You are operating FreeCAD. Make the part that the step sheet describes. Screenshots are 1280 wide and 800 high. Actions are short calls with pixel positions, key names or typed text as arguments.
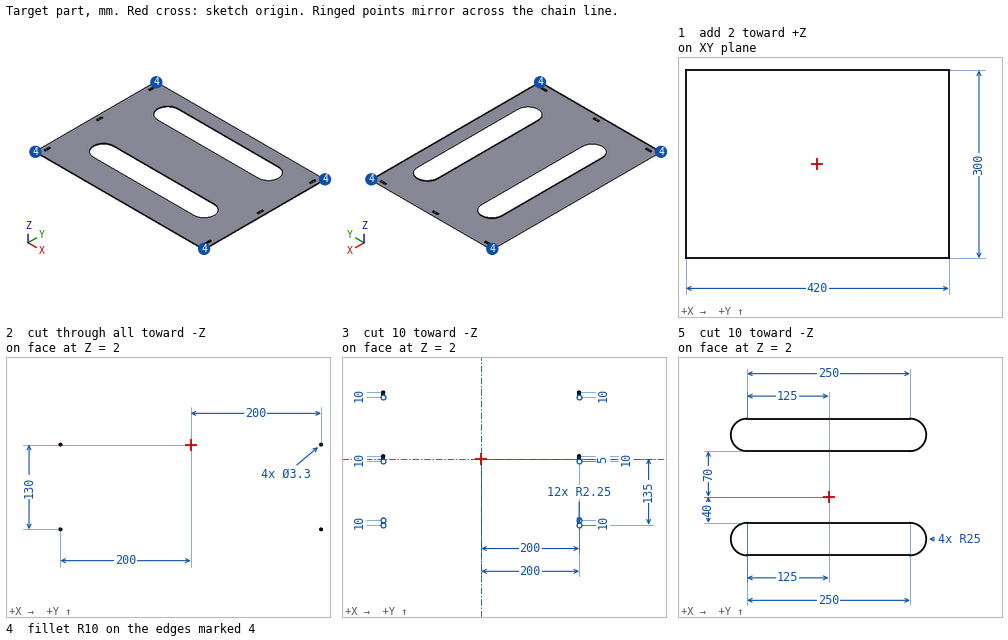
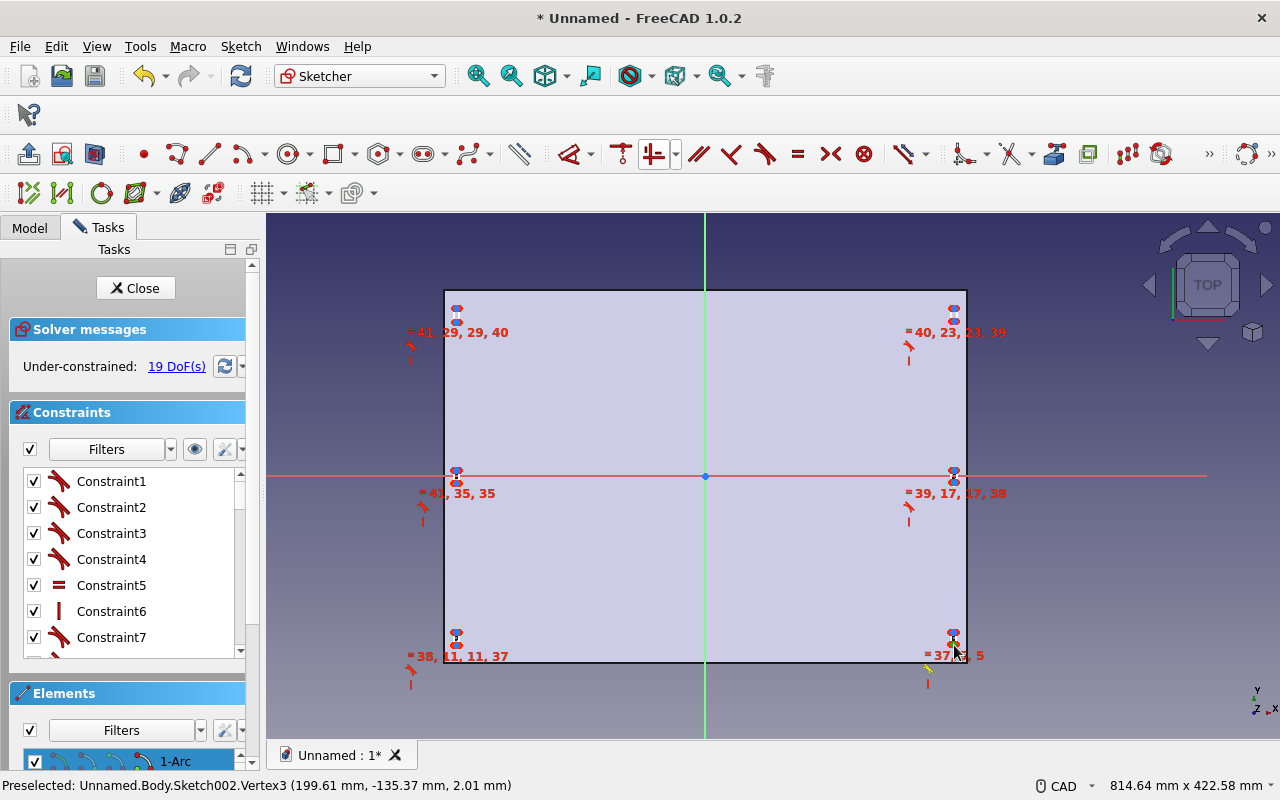
scroll(456, 645, up, 8)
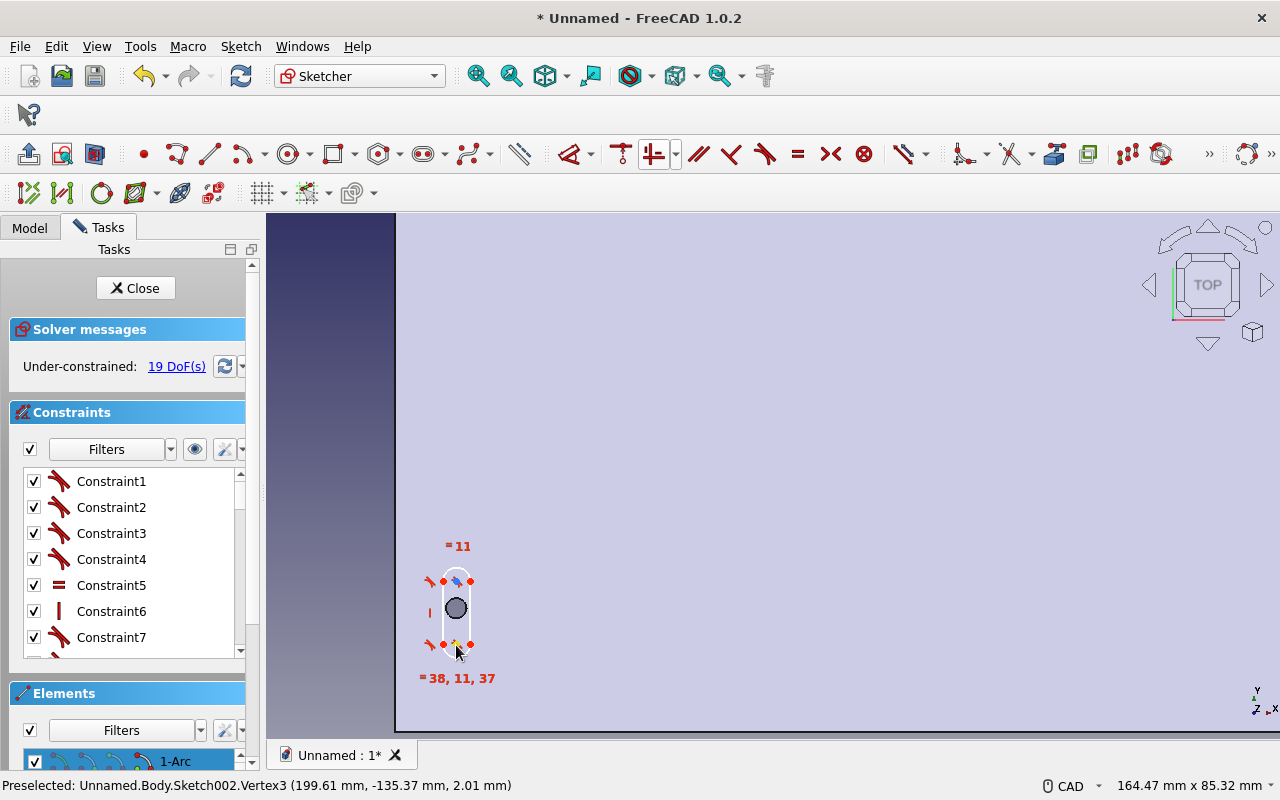
click(457, 644)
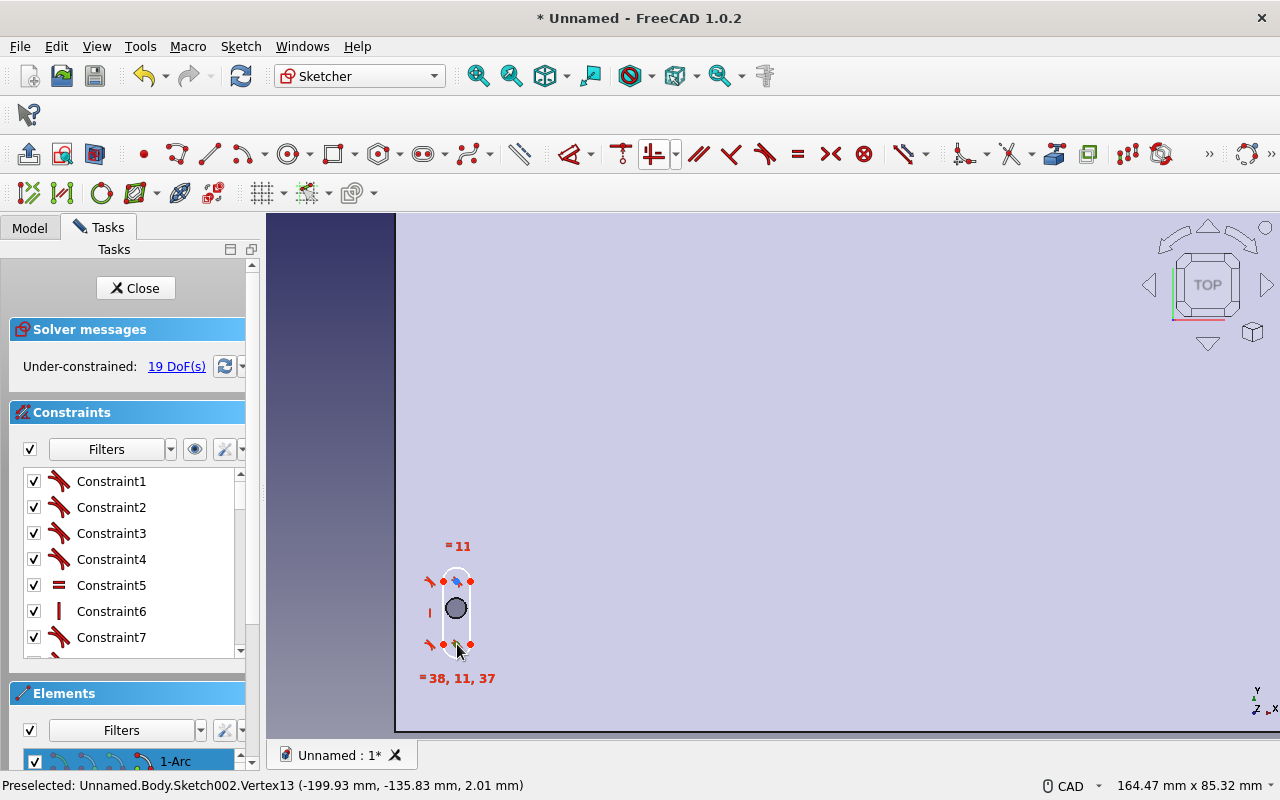
scroll(455, 645, down, 8)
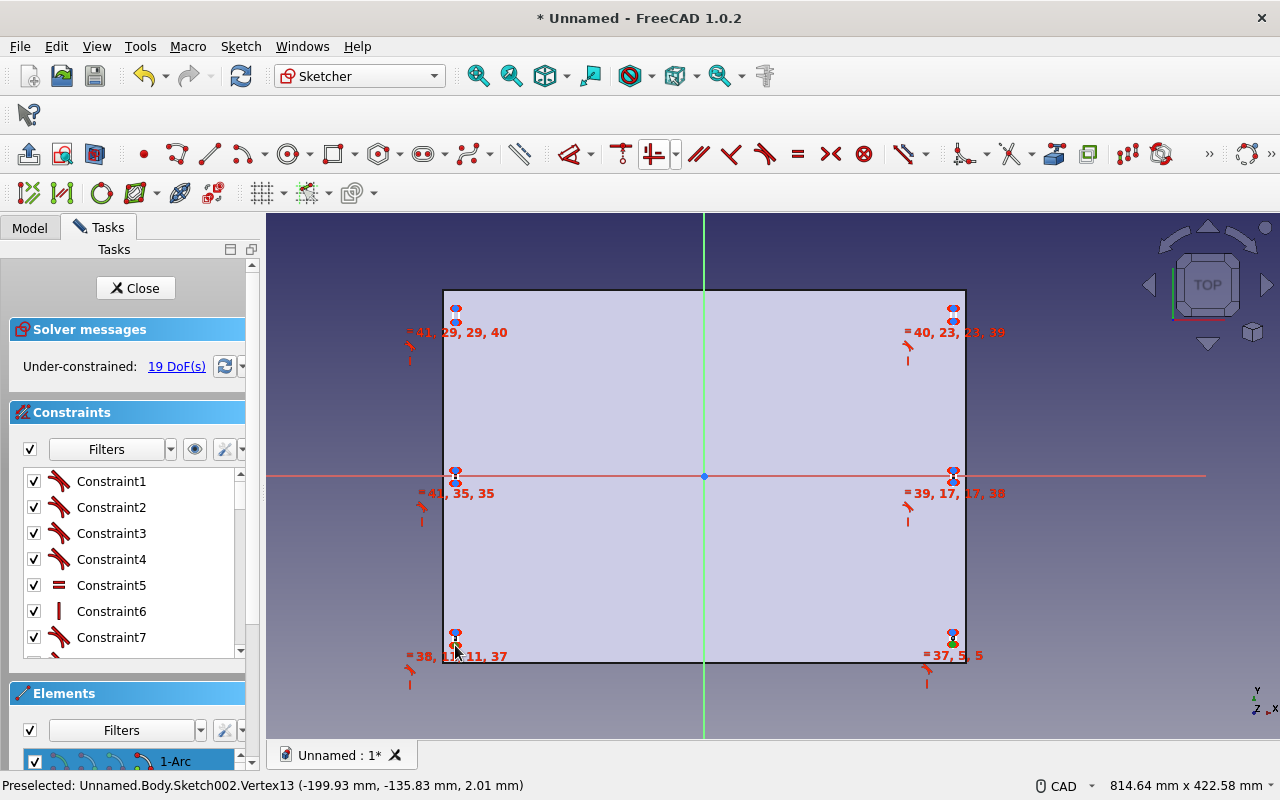
click(704, 677)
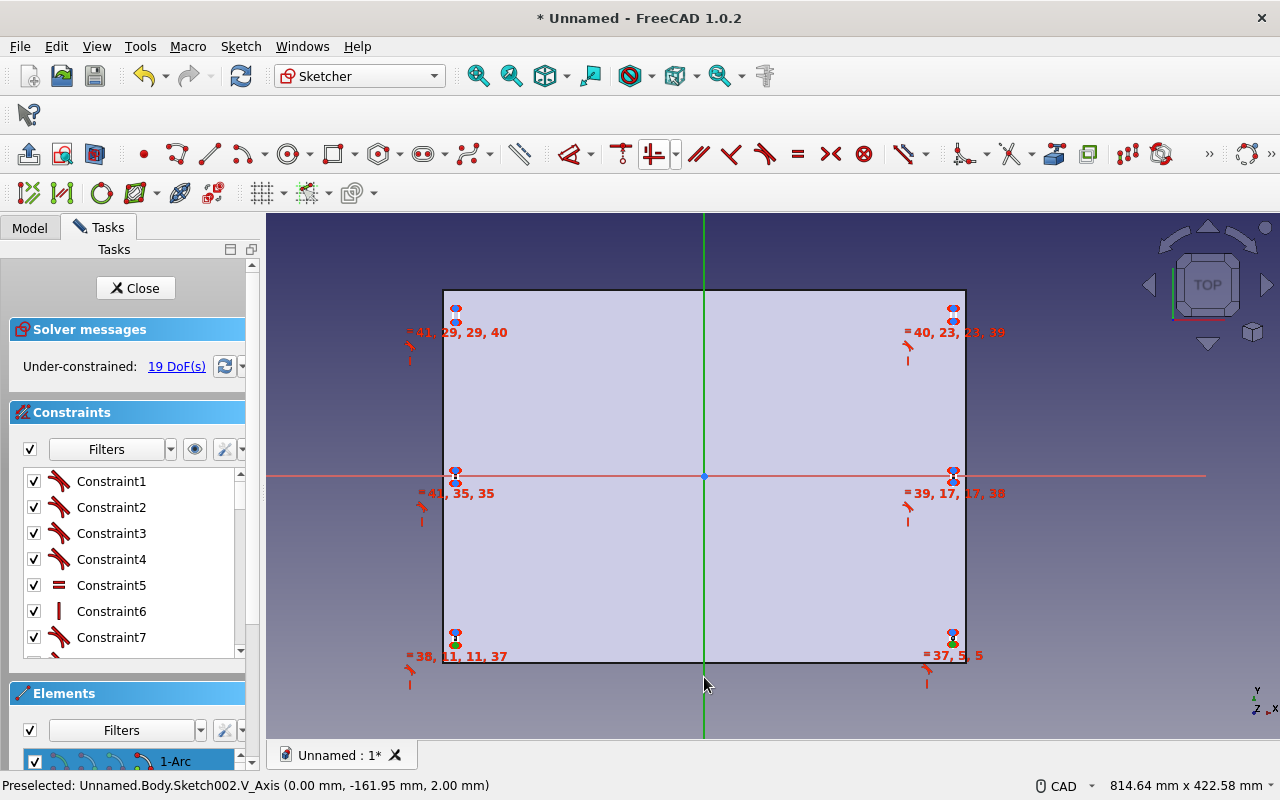
click(831, 154)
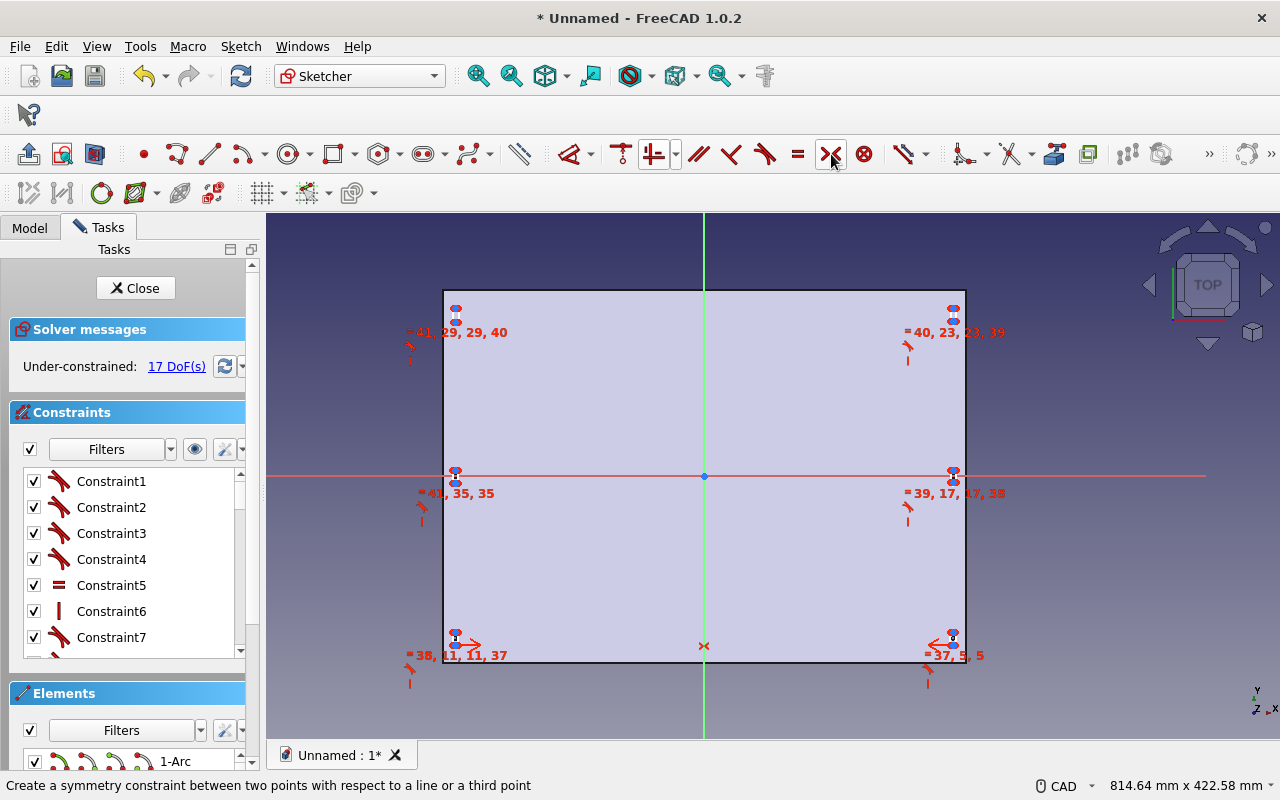
scroll(953, 633, up, 8)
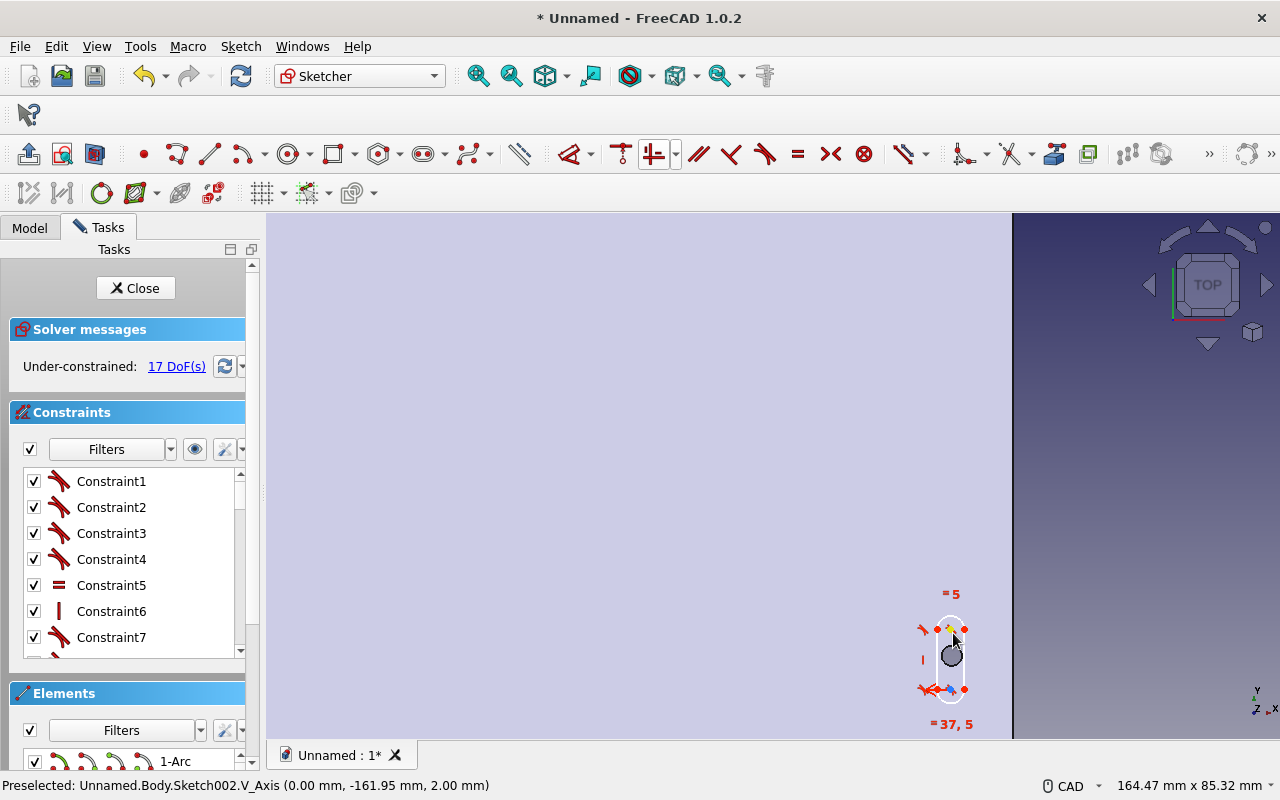
click(951, 630)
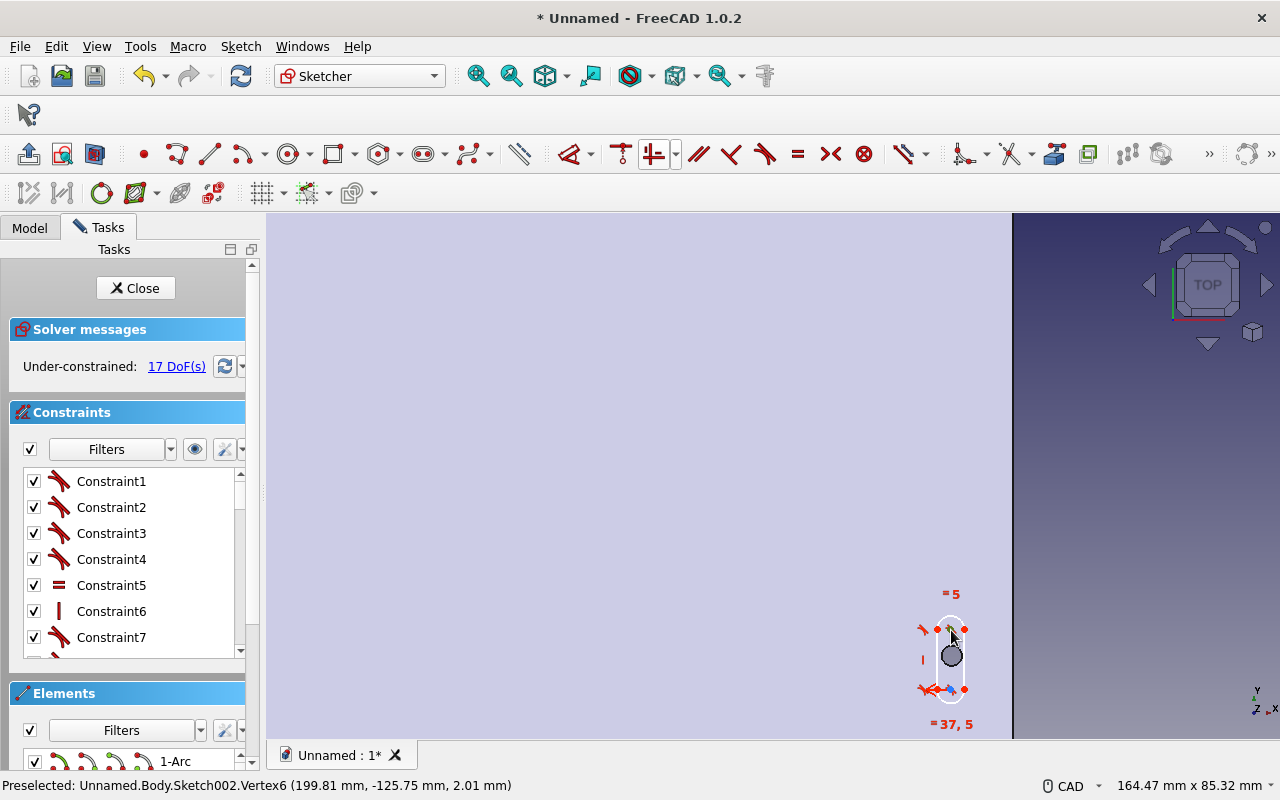
scroll(954, 633, down, 8)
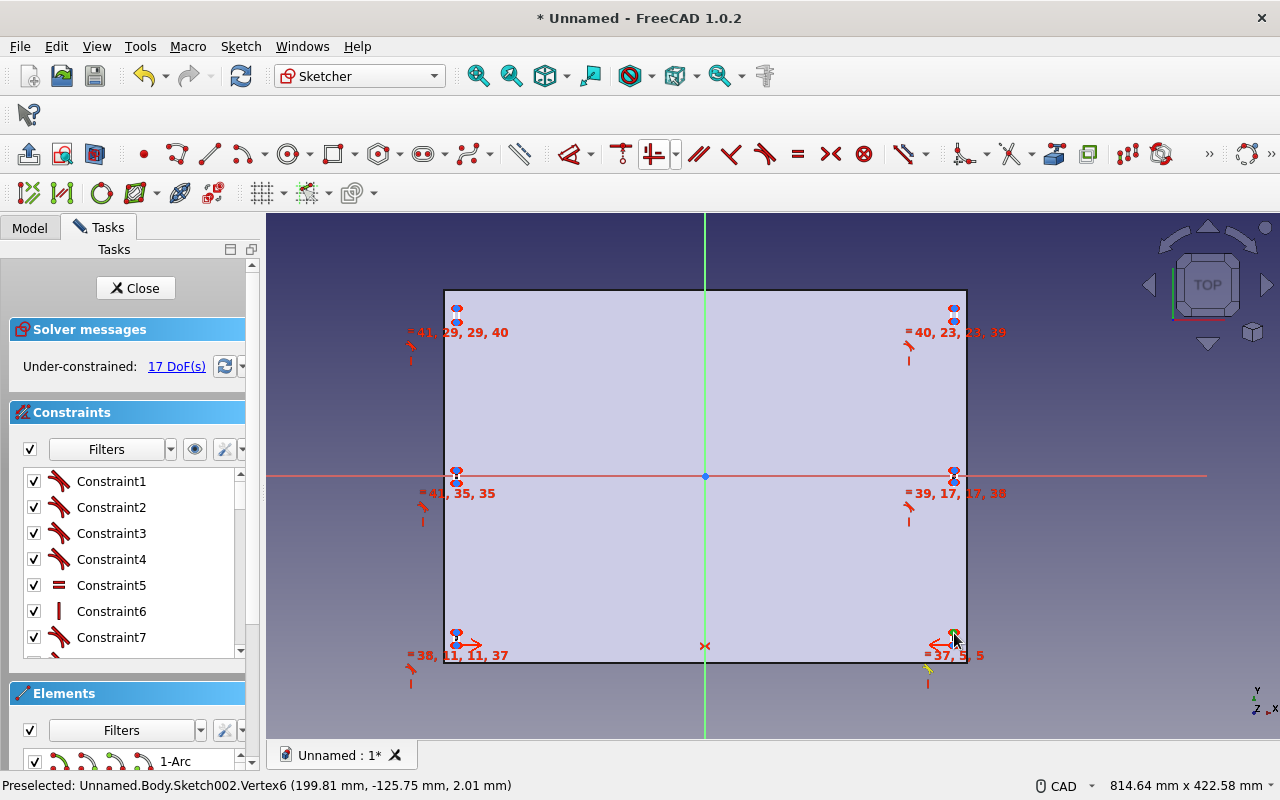
scroll(954, 322, up, 8)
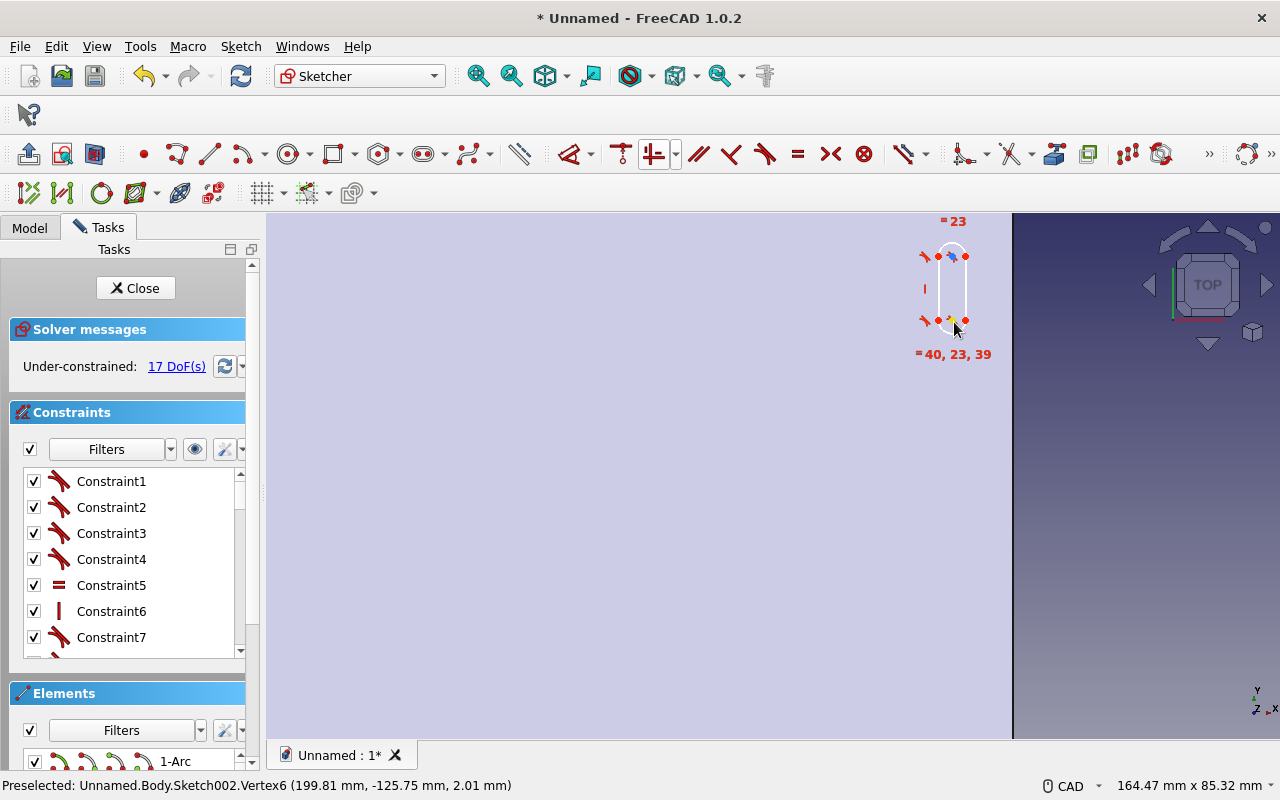
click(952, 320)